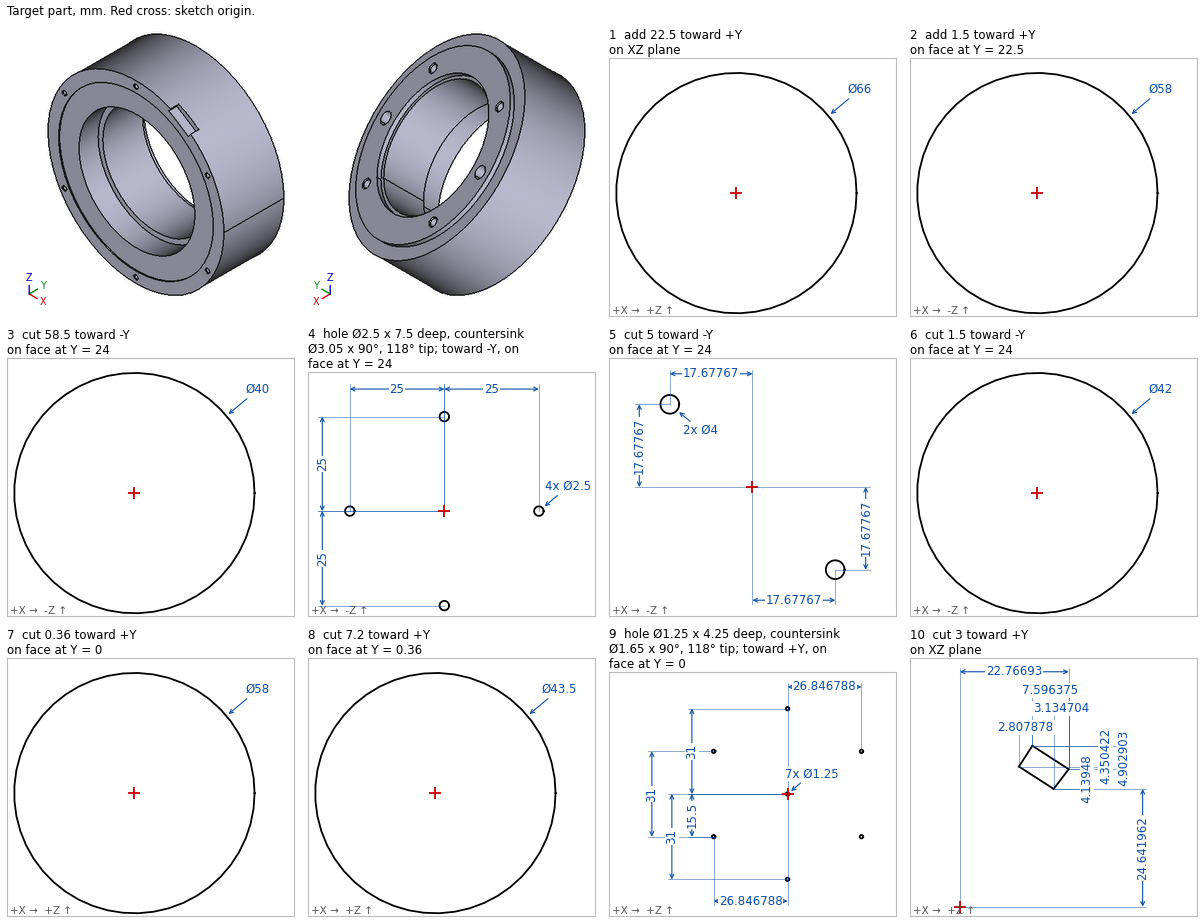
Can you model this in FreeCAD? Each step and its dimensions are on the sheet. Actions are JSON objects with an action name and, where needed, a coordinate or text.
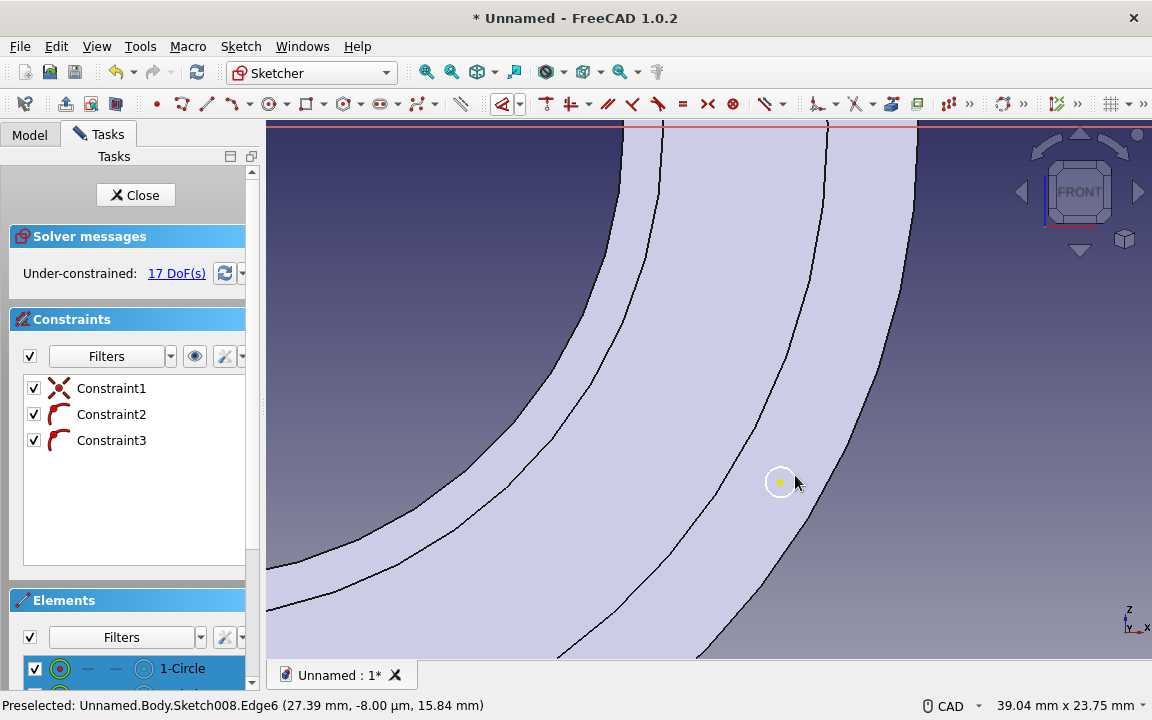
{"action": "left_click", "coordinate": [791, 472]}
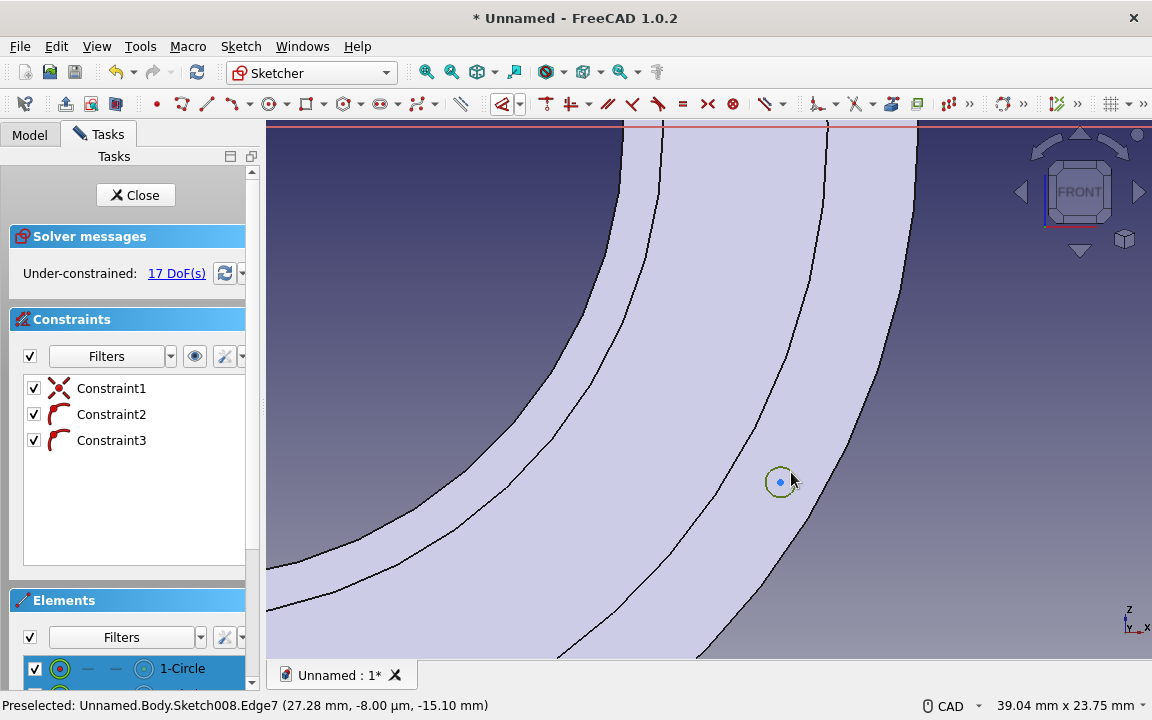
{"action": "left_click", "coordinate": [683, 104]}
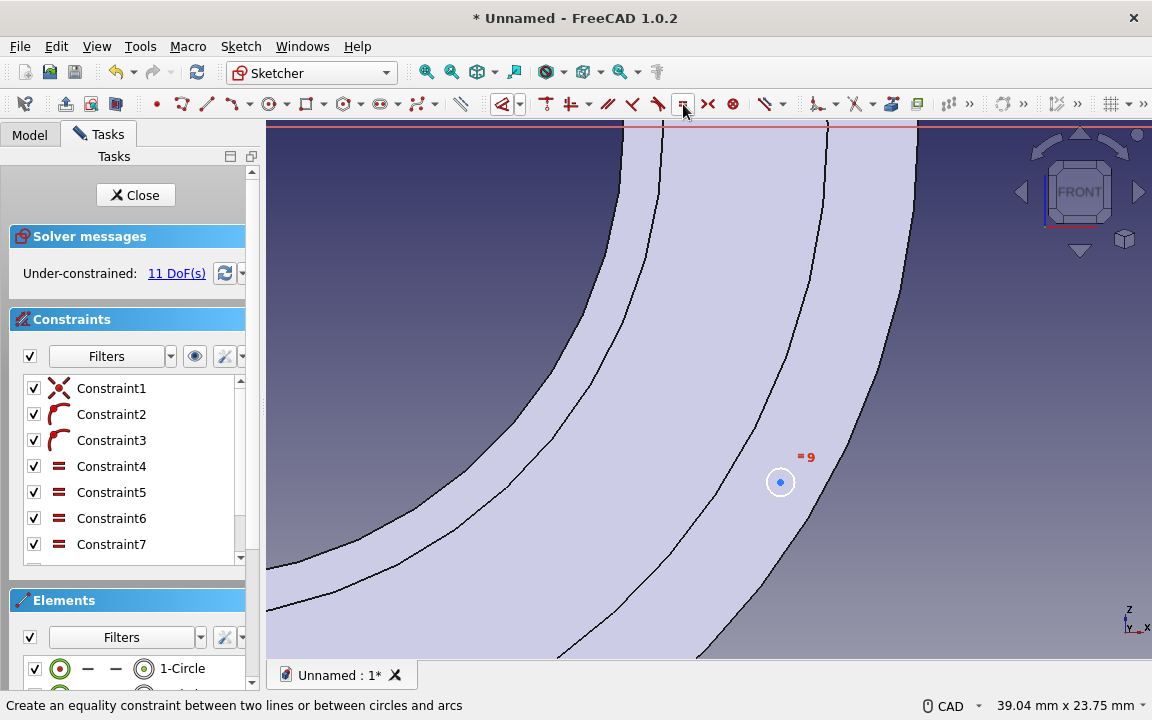
{"action": "scroll", "coordinate": [795, 475], "scroll_direction": "down", "scroll_amount": 7}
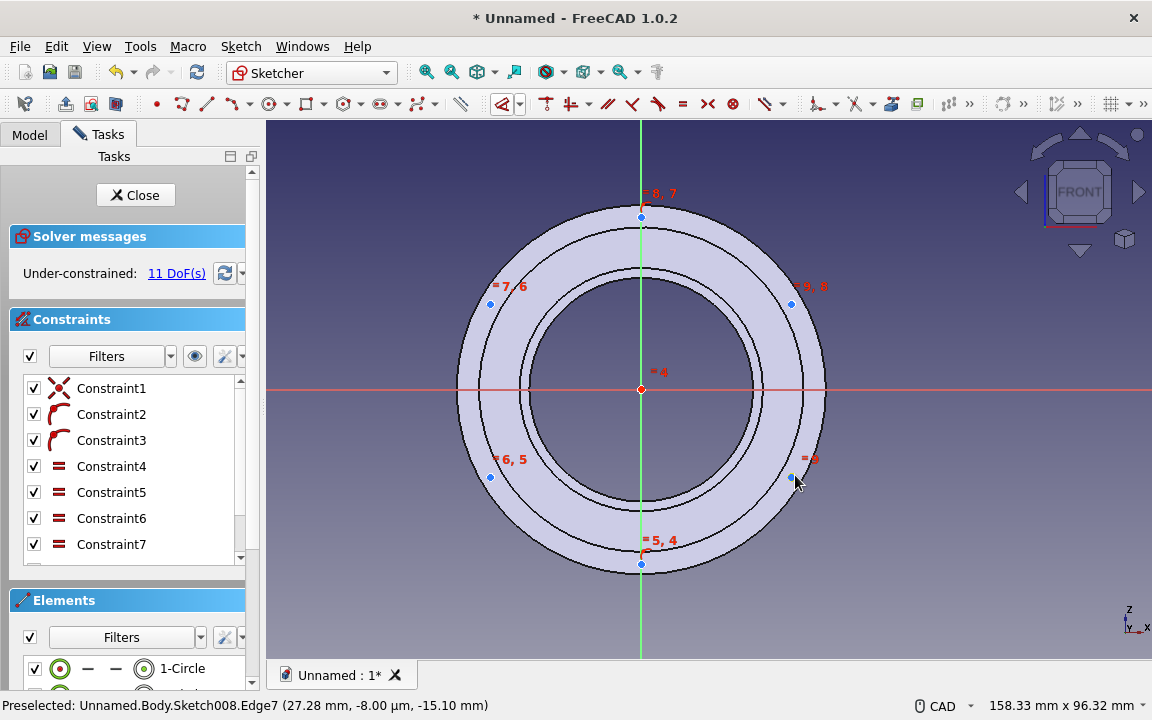
{"action": "left_click", "coordinate": [491, 477]}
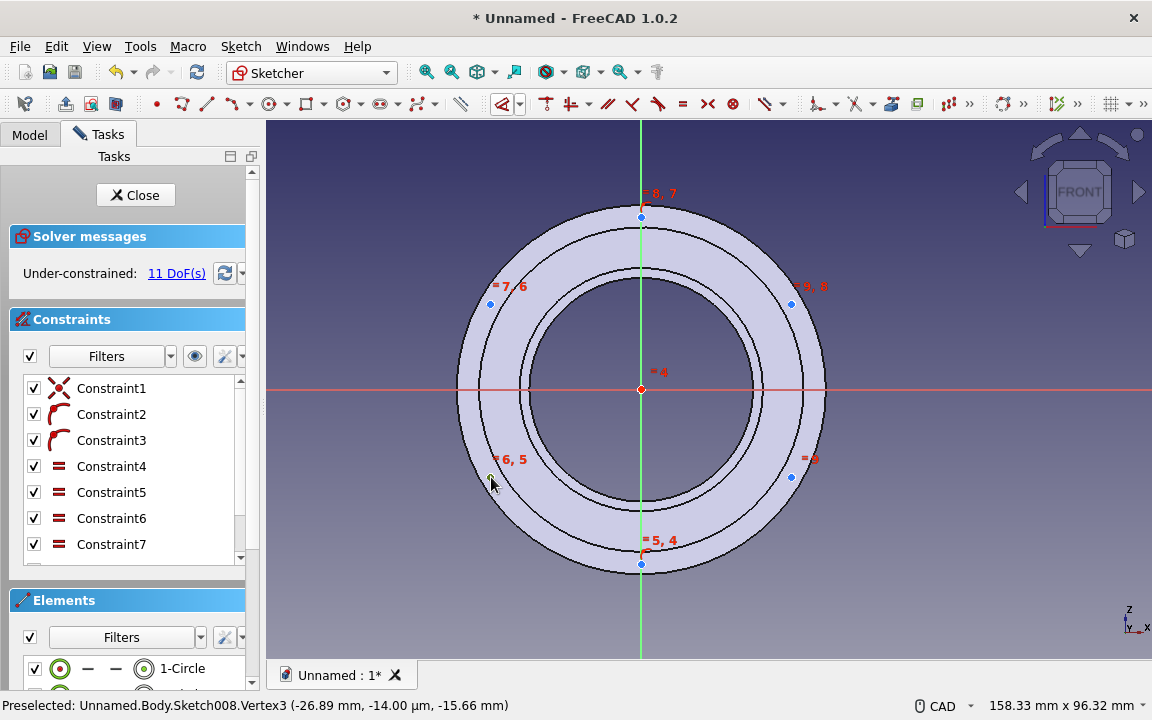
{"action": "left_click", "coordinate": [491, 304]}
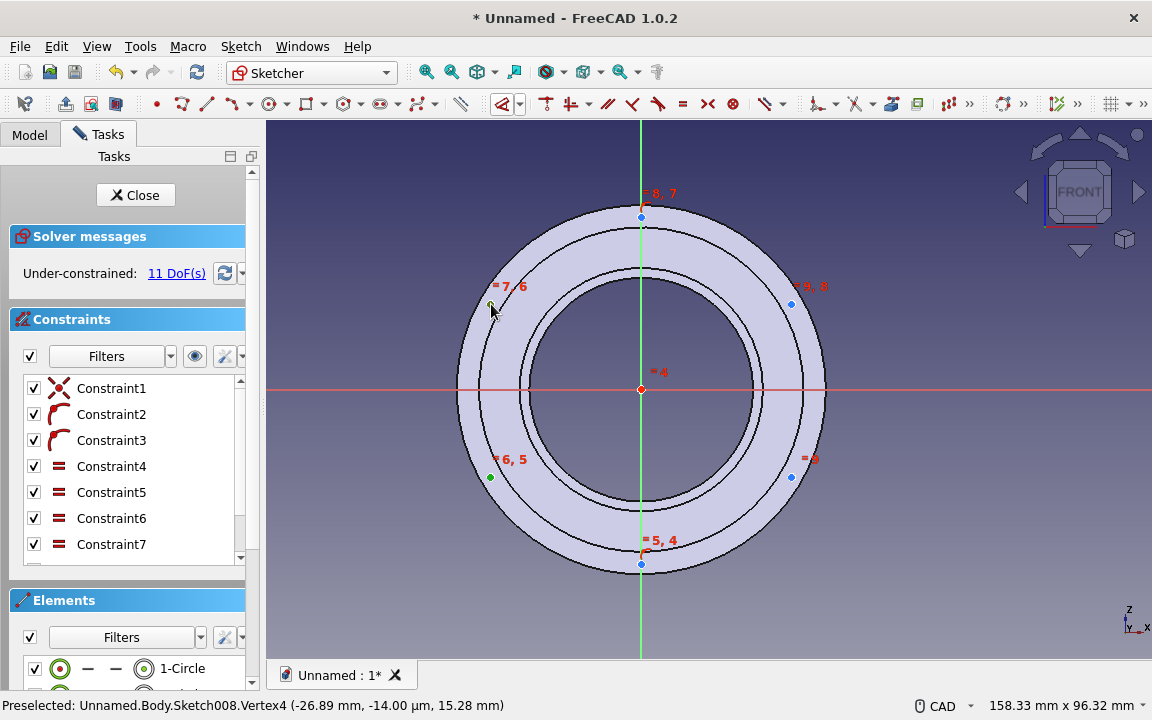
{"action": "left_click", "coordinate": [588, 104]}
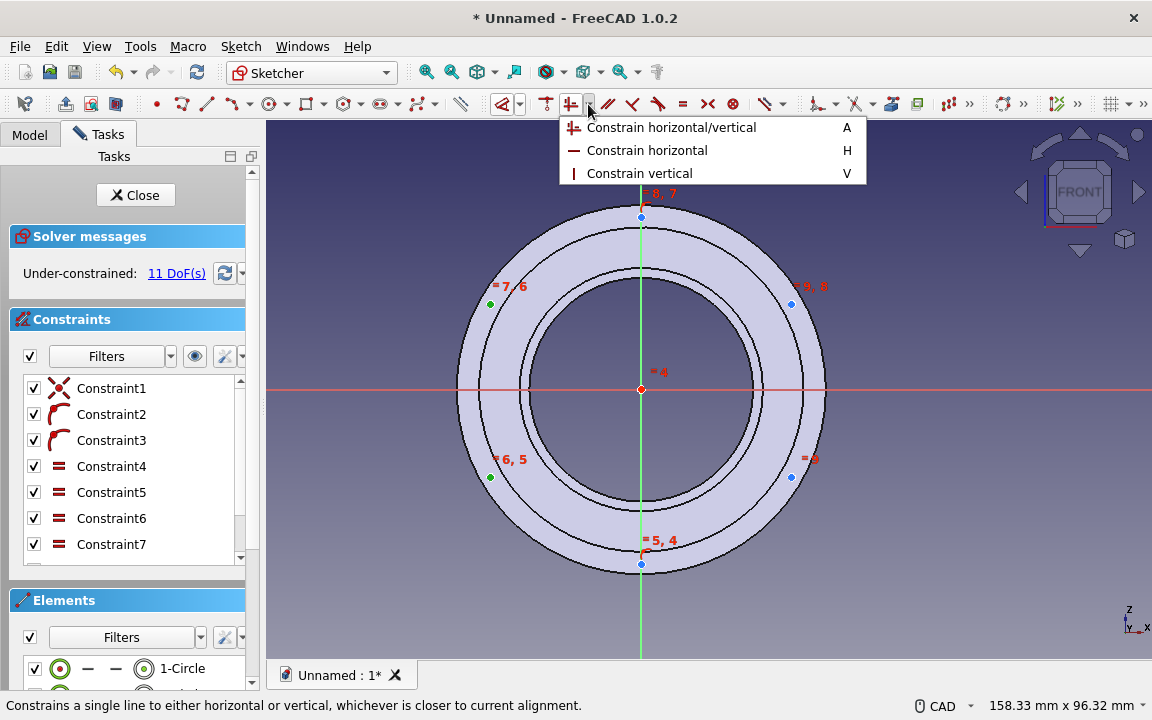
{"action": "left_click", "coordinate": [713, 174]}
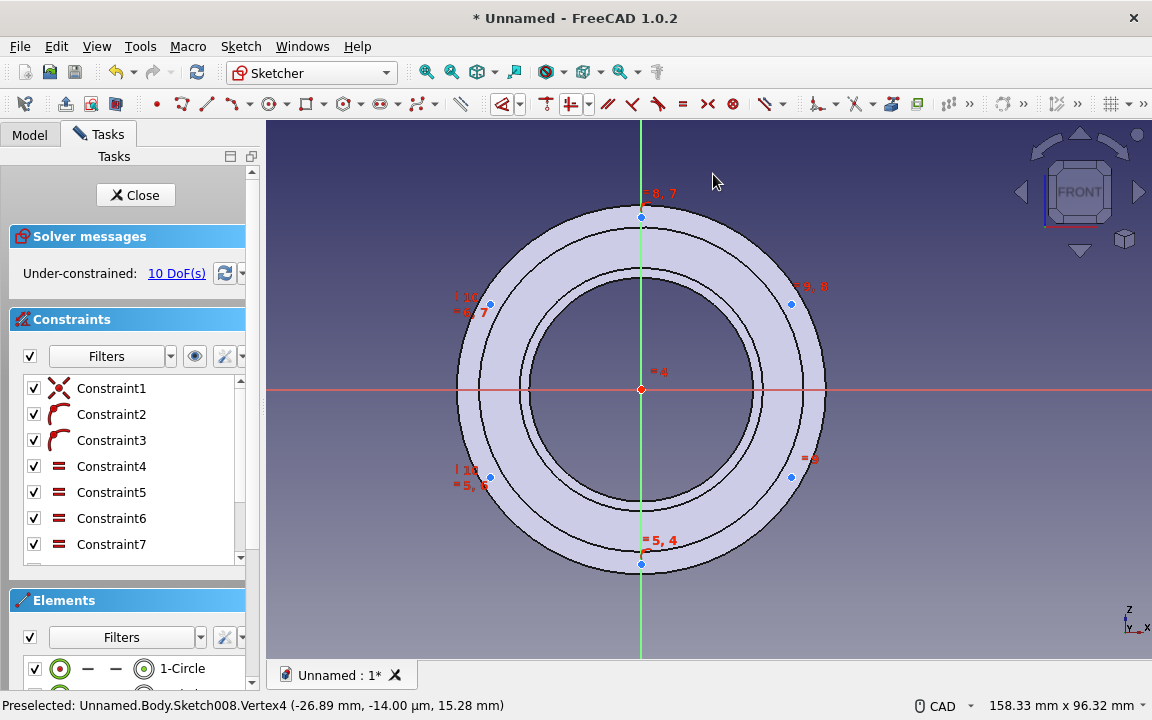
{"action": "left_click", "coordinate": [491, 304]}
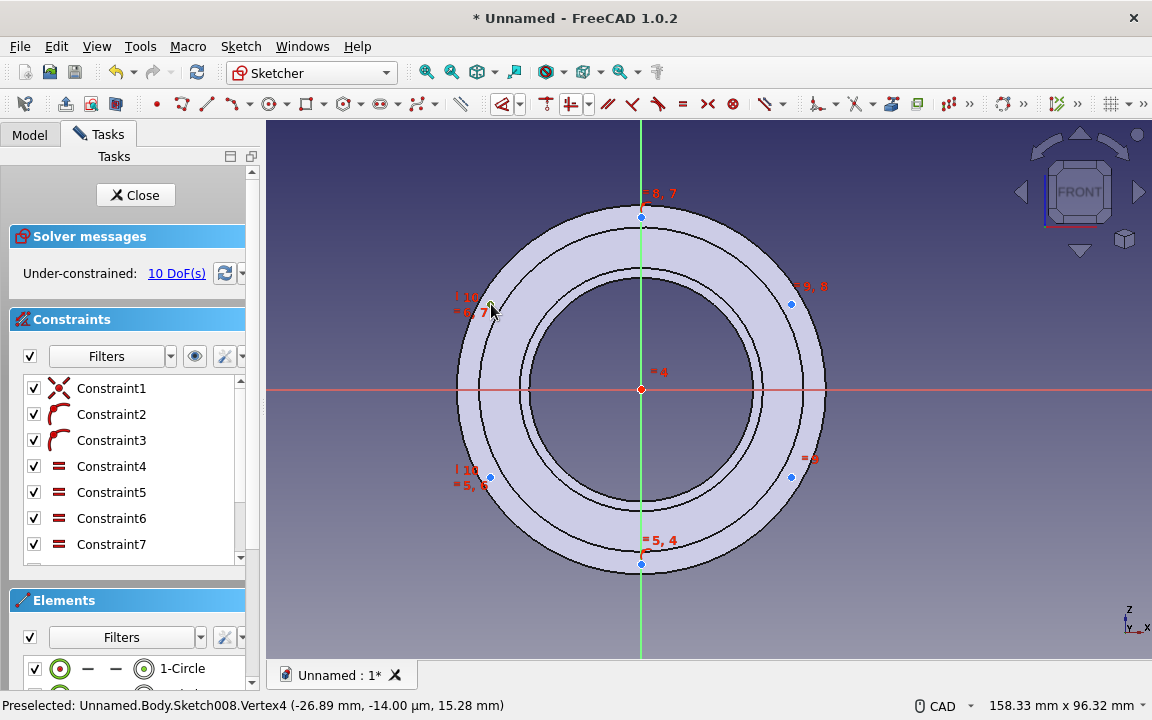
{"action": "left_click", "coordinate": [792, 304]}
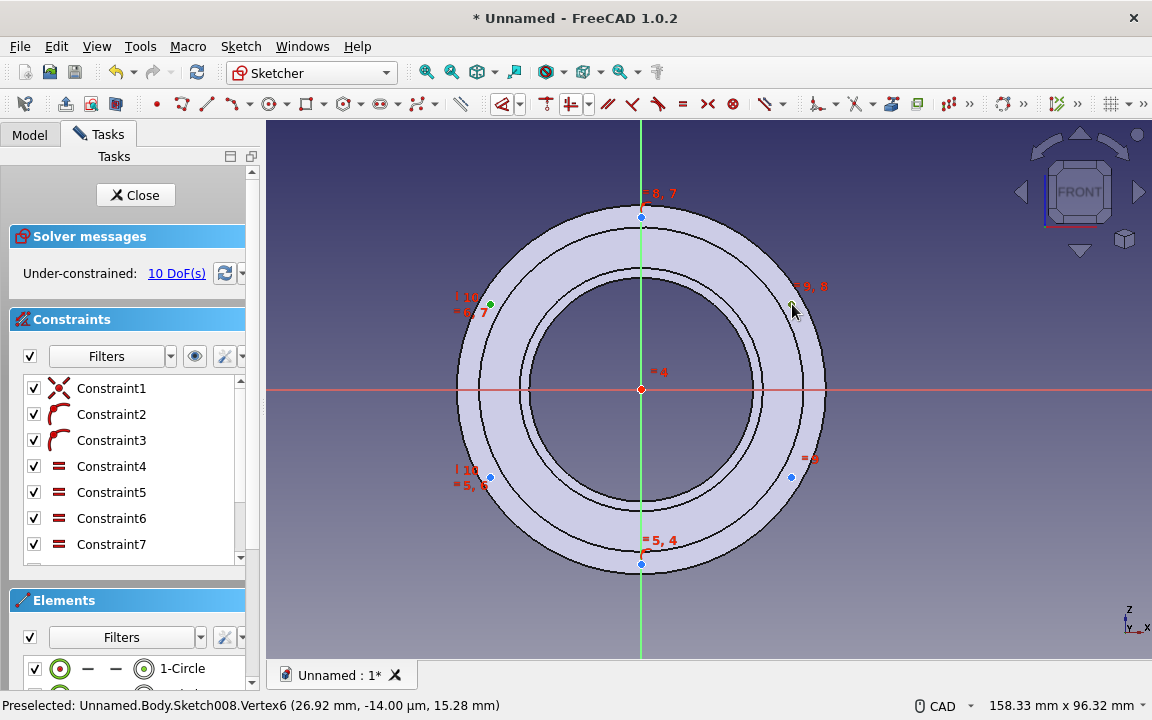
{"action": "key", "text": "h"}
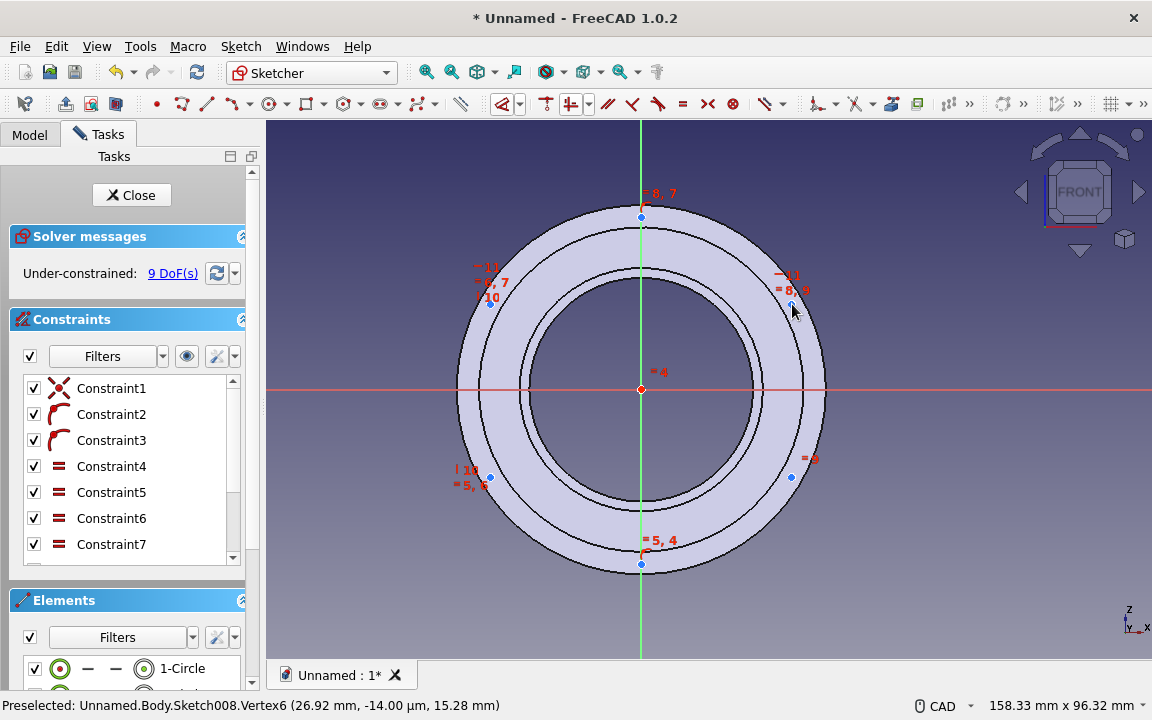
{"action": "left_click", "coordinate": [792, 304]}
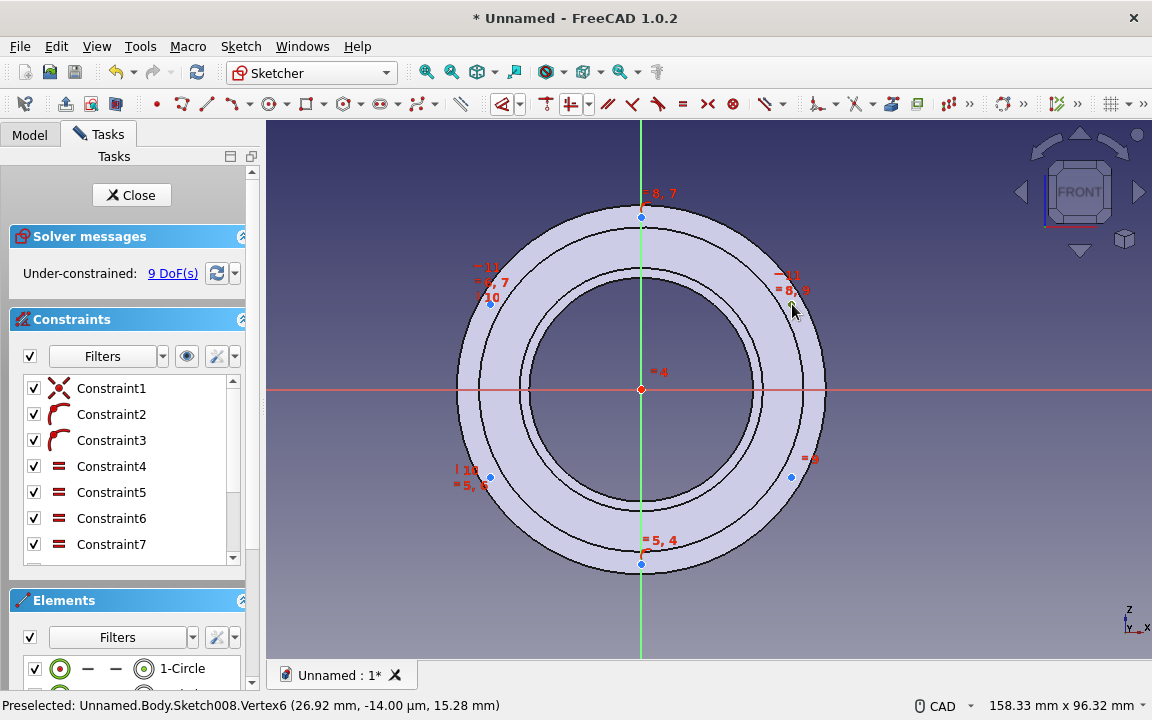
{"action": "left_click", "coordinate": [792, 477]}